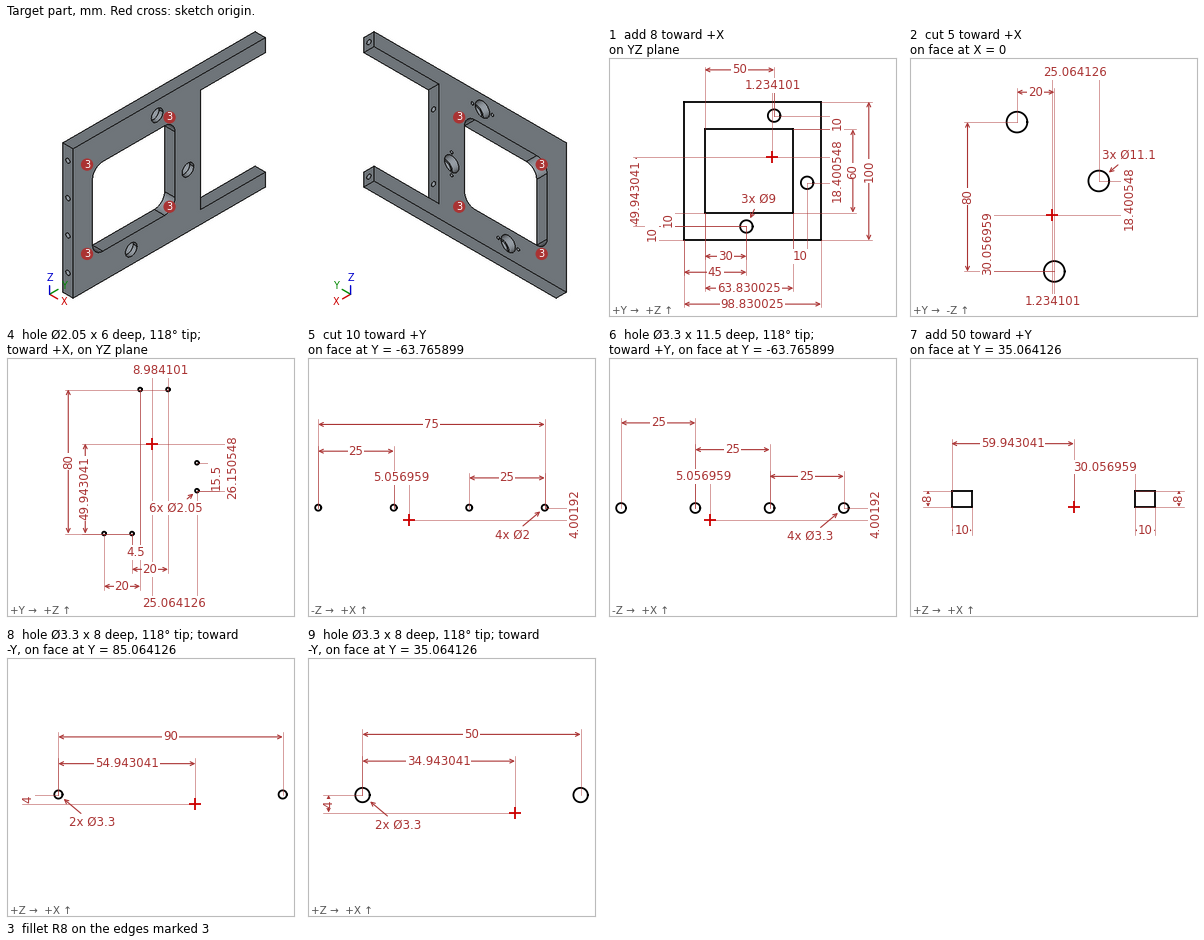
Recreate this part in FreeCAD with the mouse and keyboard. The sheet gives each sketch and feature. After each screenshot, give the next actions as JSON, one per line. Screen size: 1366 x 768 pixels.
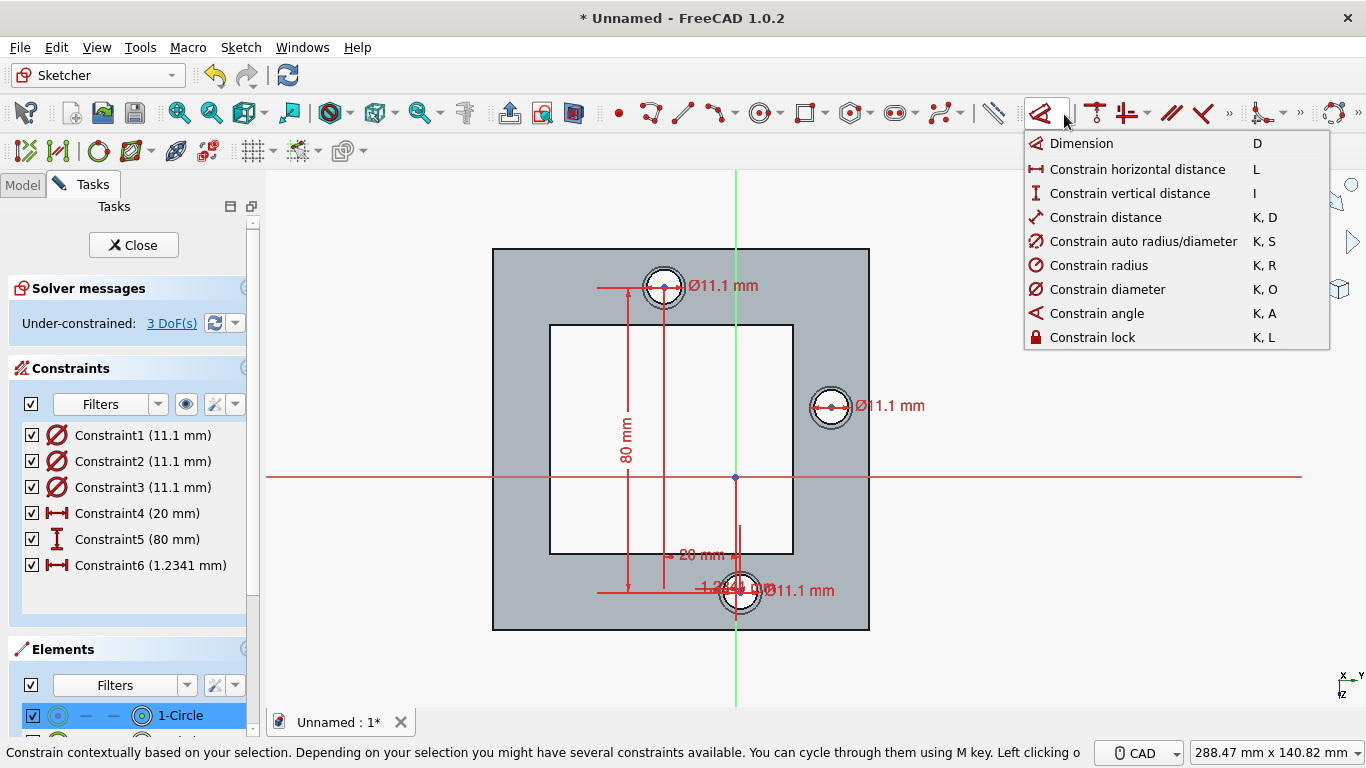
{"action": "left_click", "coordinate": [1177, 169]}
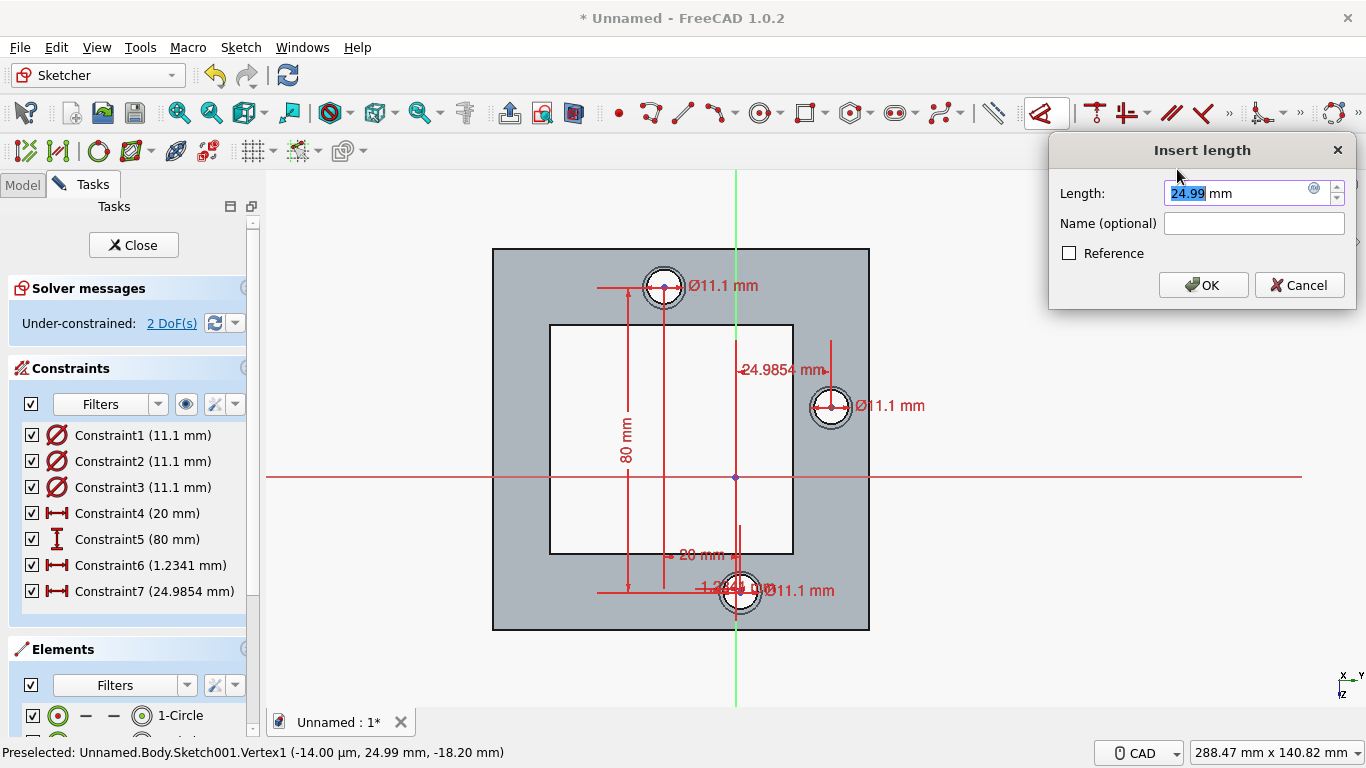
{"action": "type", "text": "25.064126"}
{"action": "key", "text": "Return"}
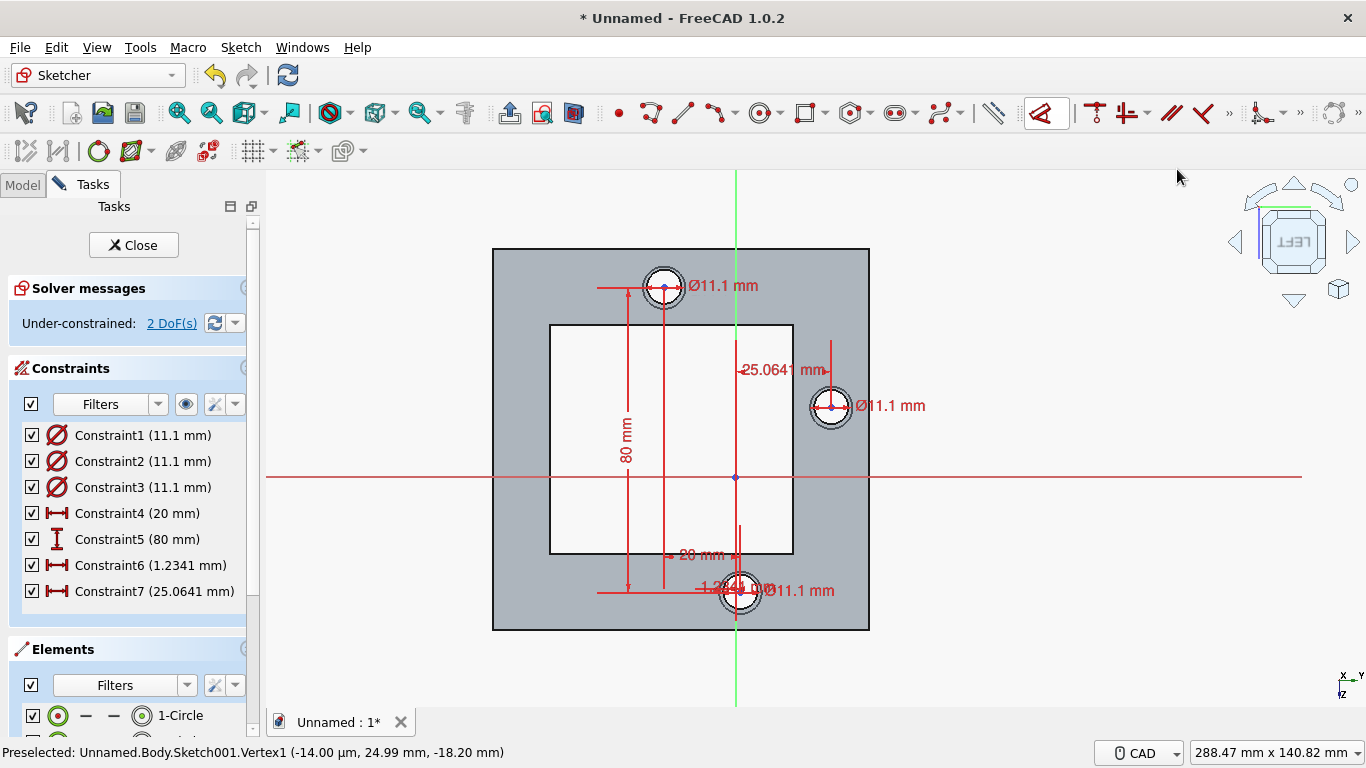
{"action": "left_click", "coordinate": [831, 408]}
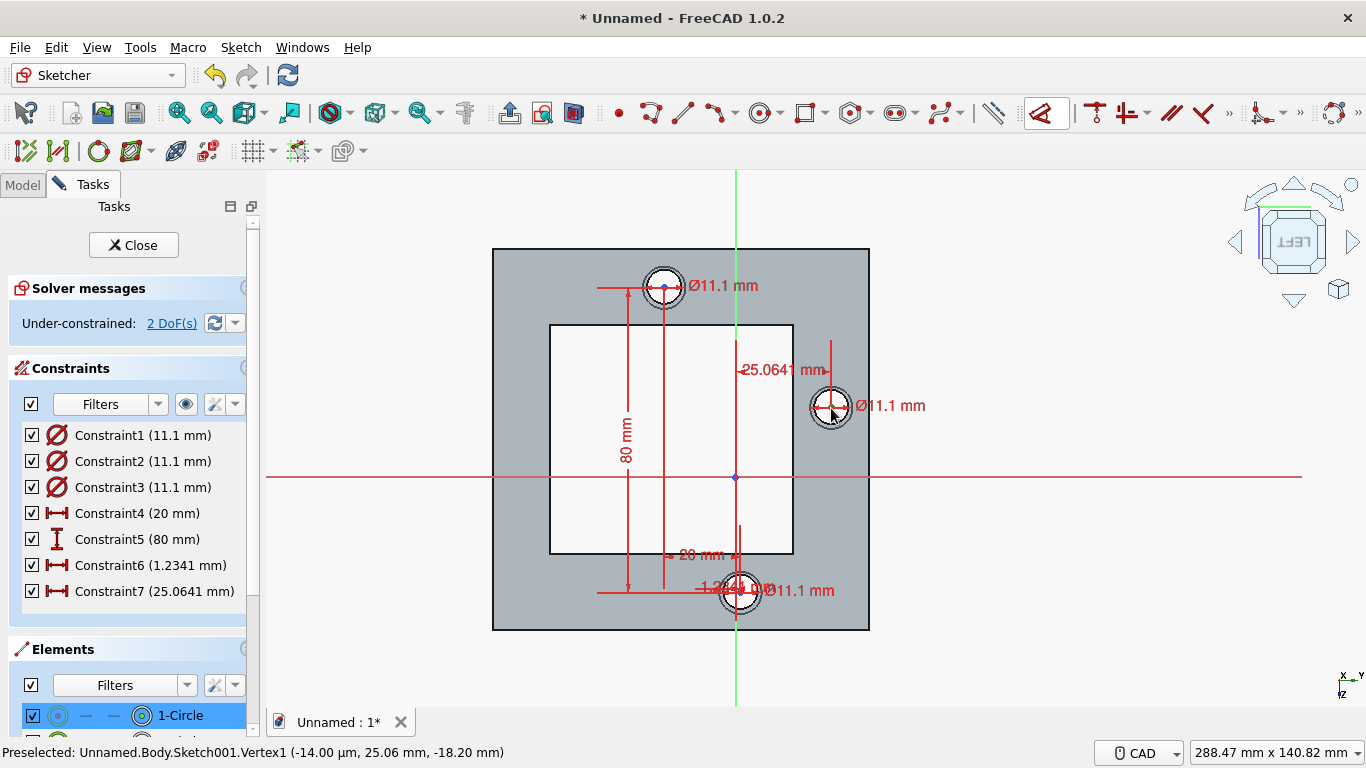
{"action": "key", "text": "i"}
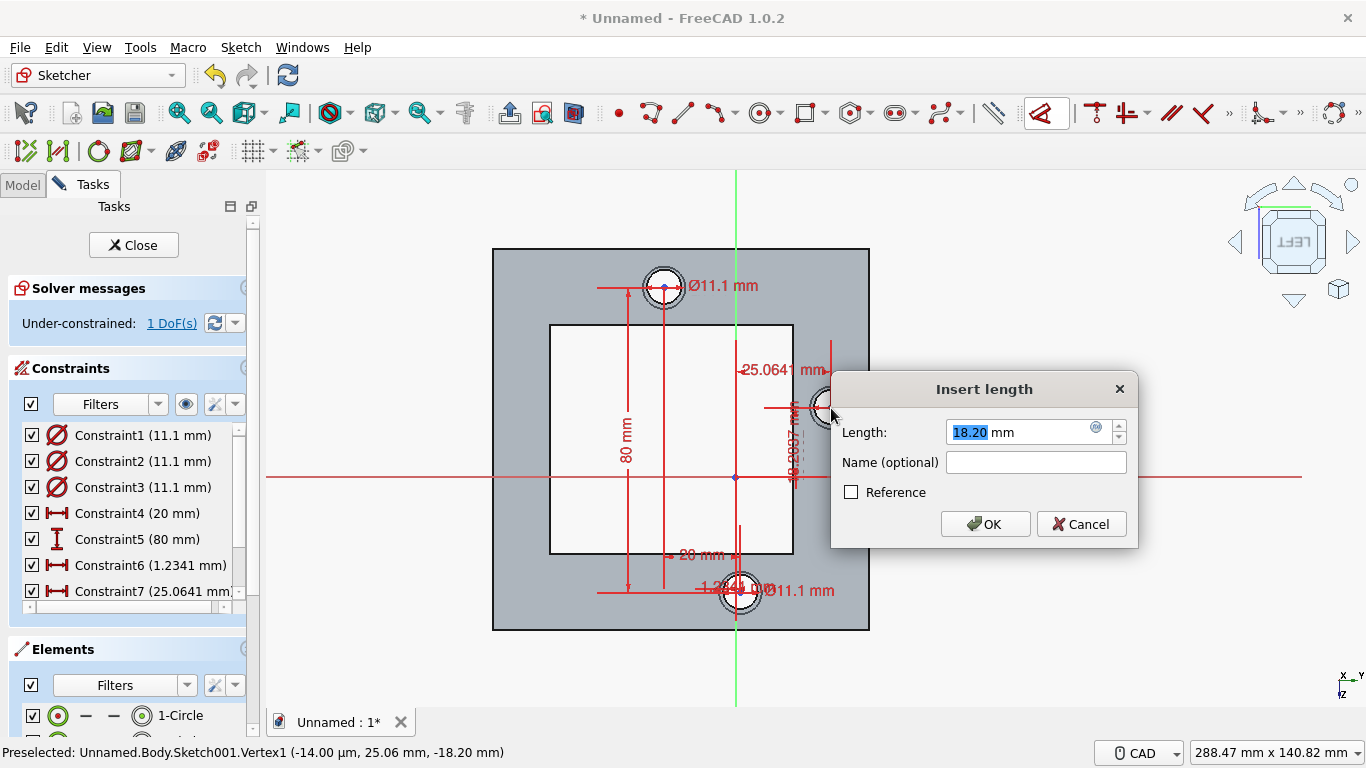
{"action": "type", "text": "18.400548"}
{"action": "key", "text": "Return"}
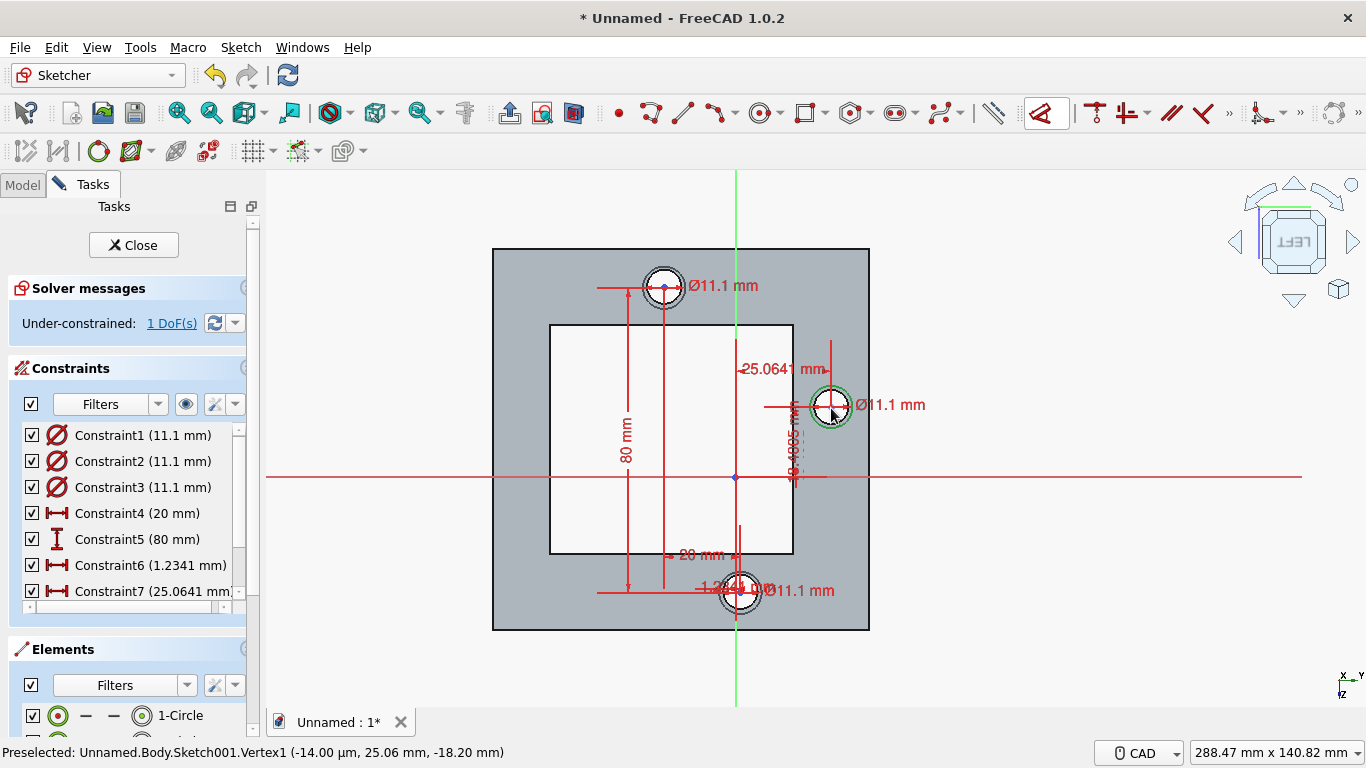
{"action": "left_click", "coordinate": [740, 593]}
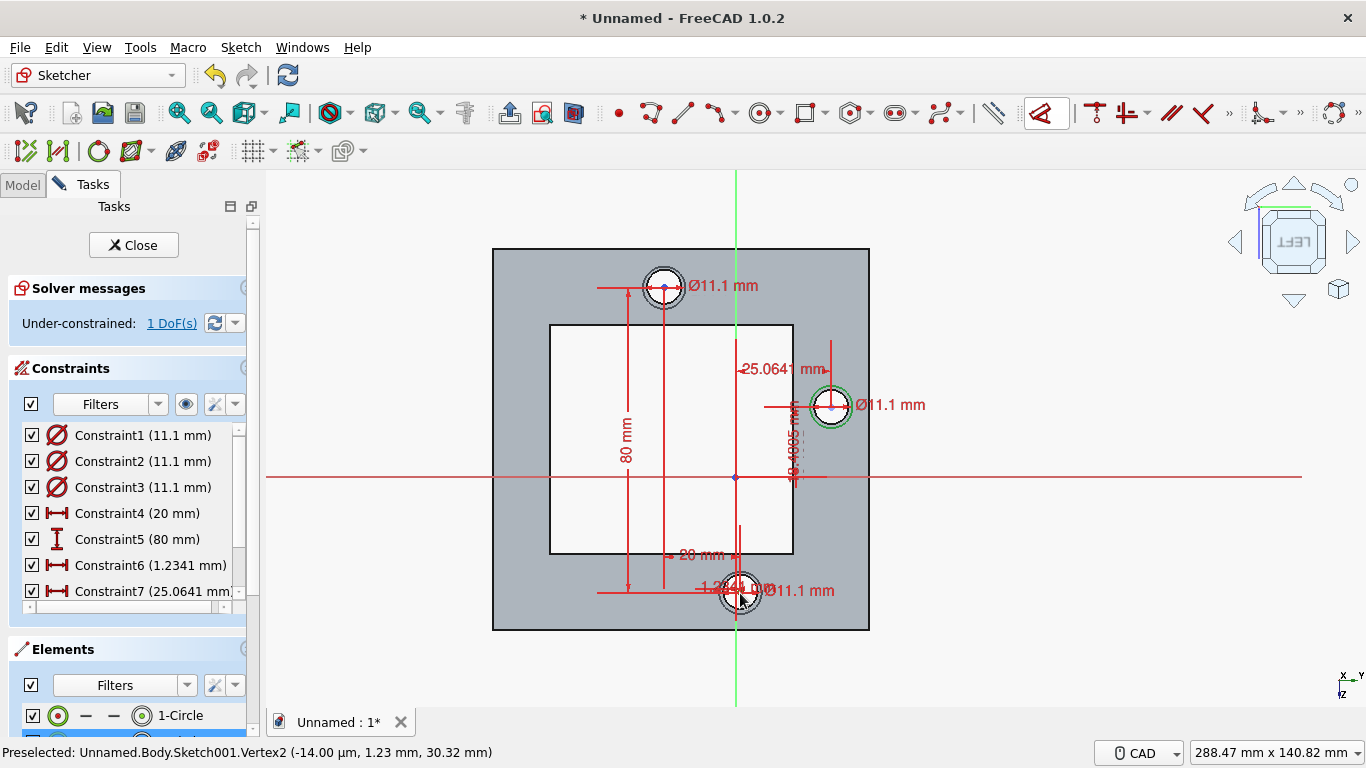
{"action": "left_click", "coordinate": [1064, 114]}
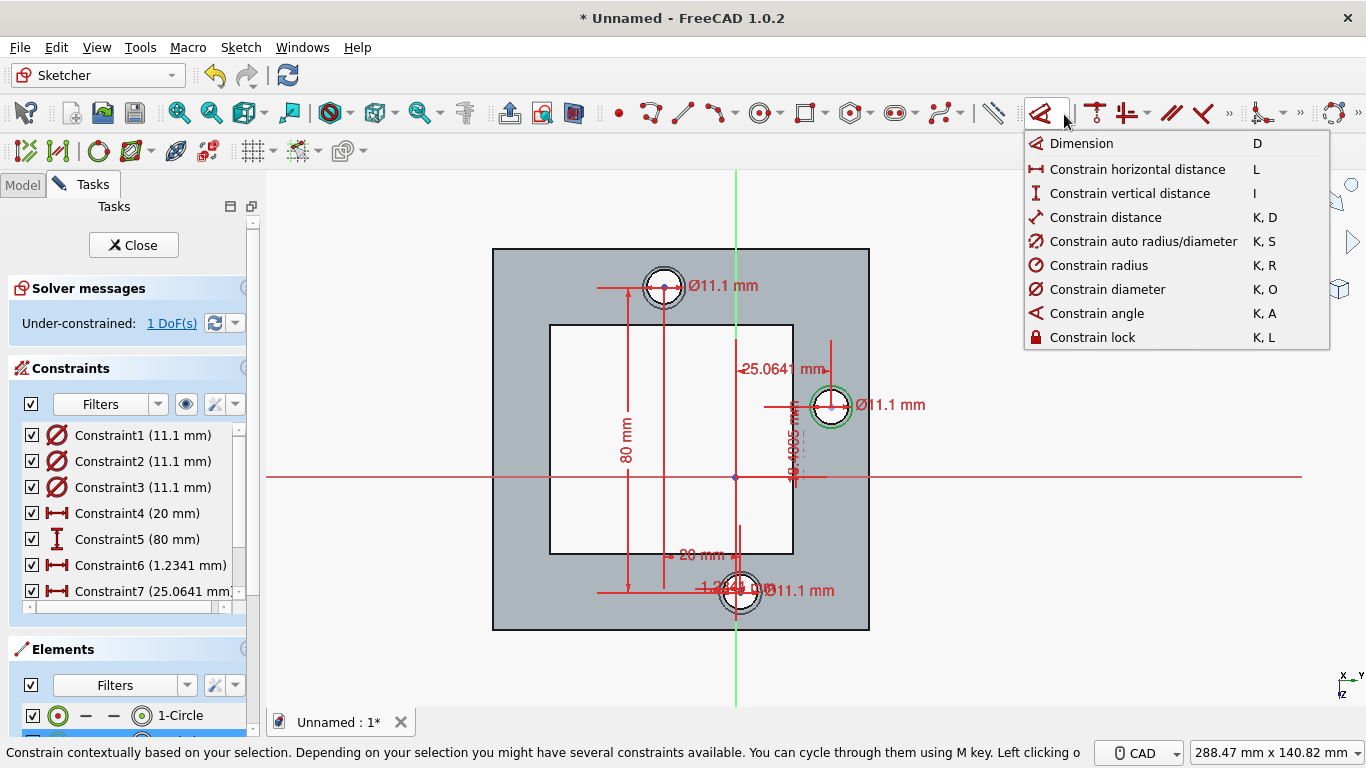
{"action": "left_click", "coordinate": [1177, 193]}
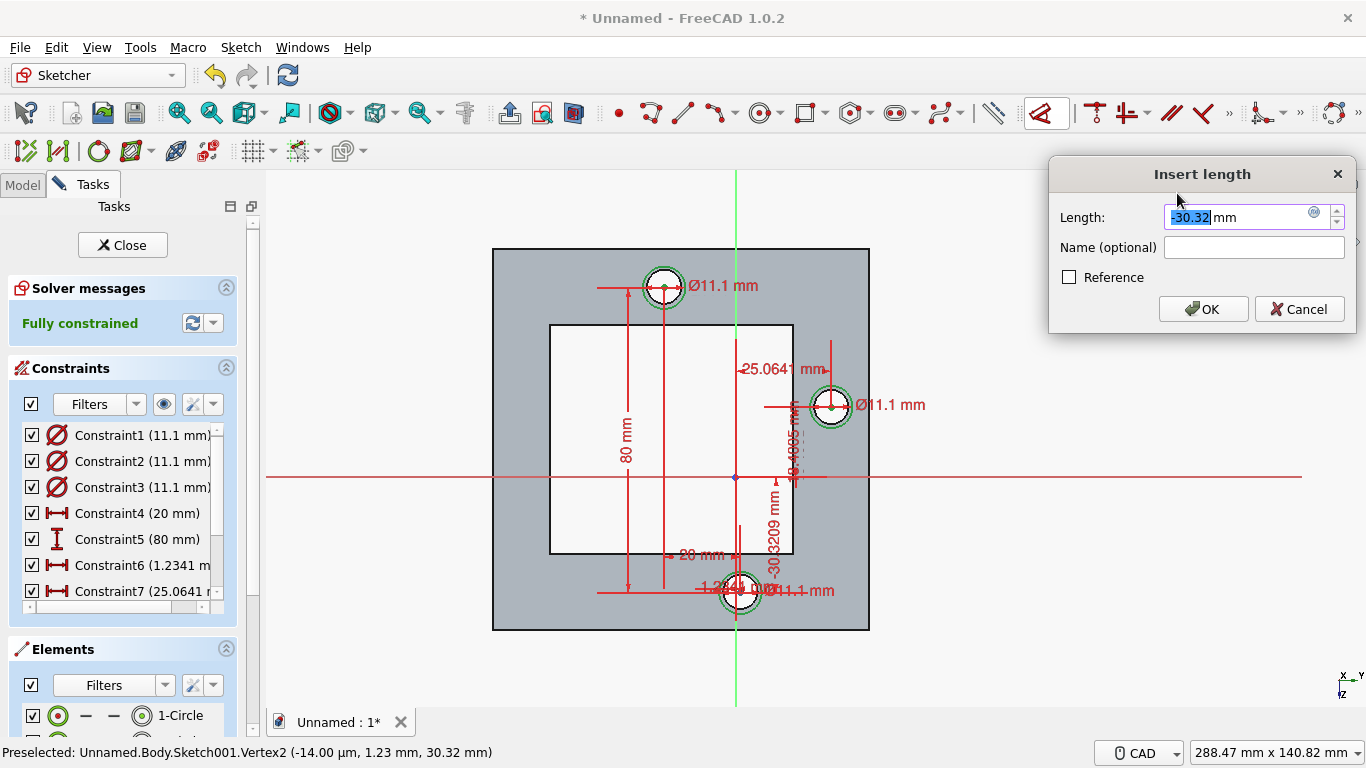
{"action": "type", "text": "-30.056959"}
{"action": "key", "text": "Return"}